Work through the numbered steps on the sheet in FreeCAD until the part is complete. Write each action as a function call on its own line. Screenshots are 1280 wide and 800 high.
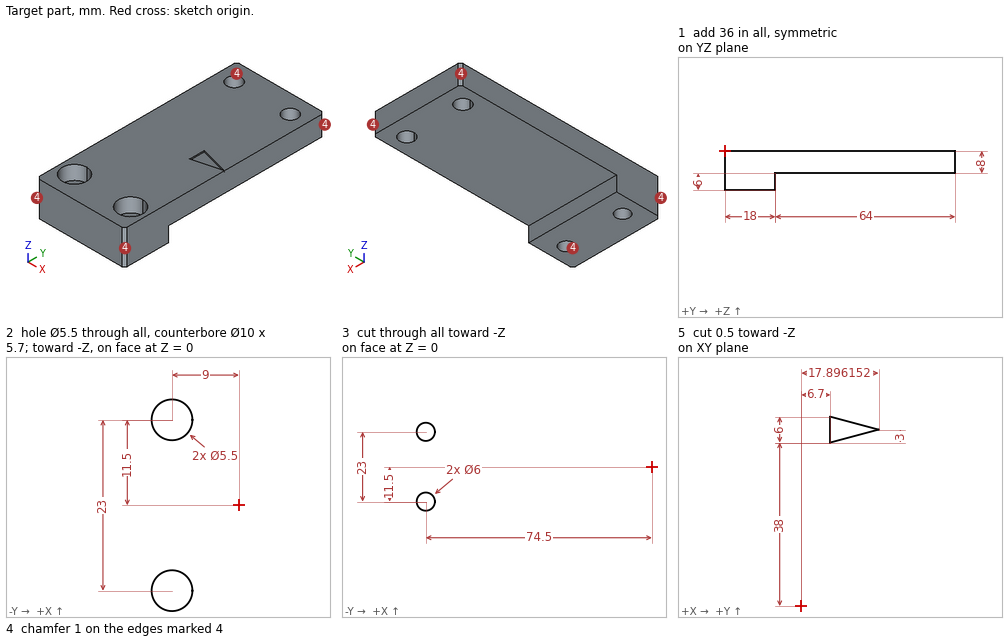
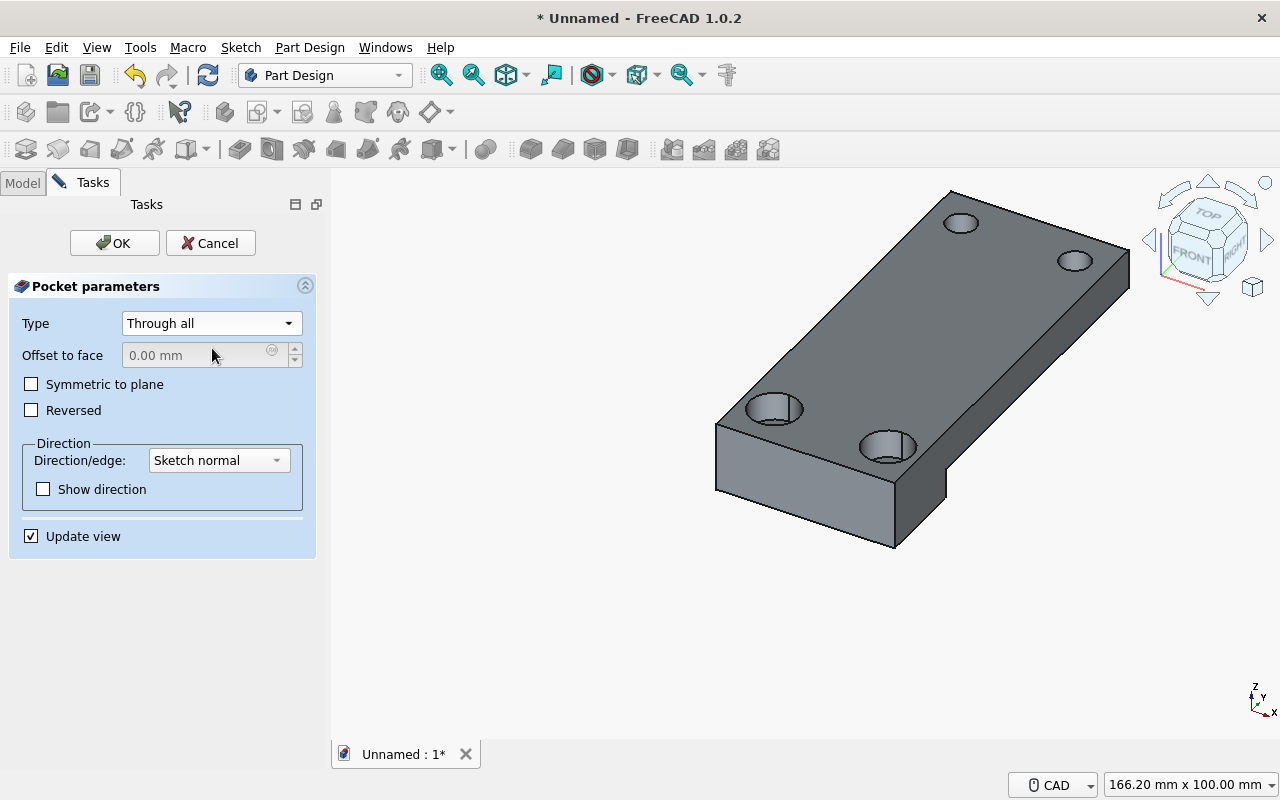
click(115, 243)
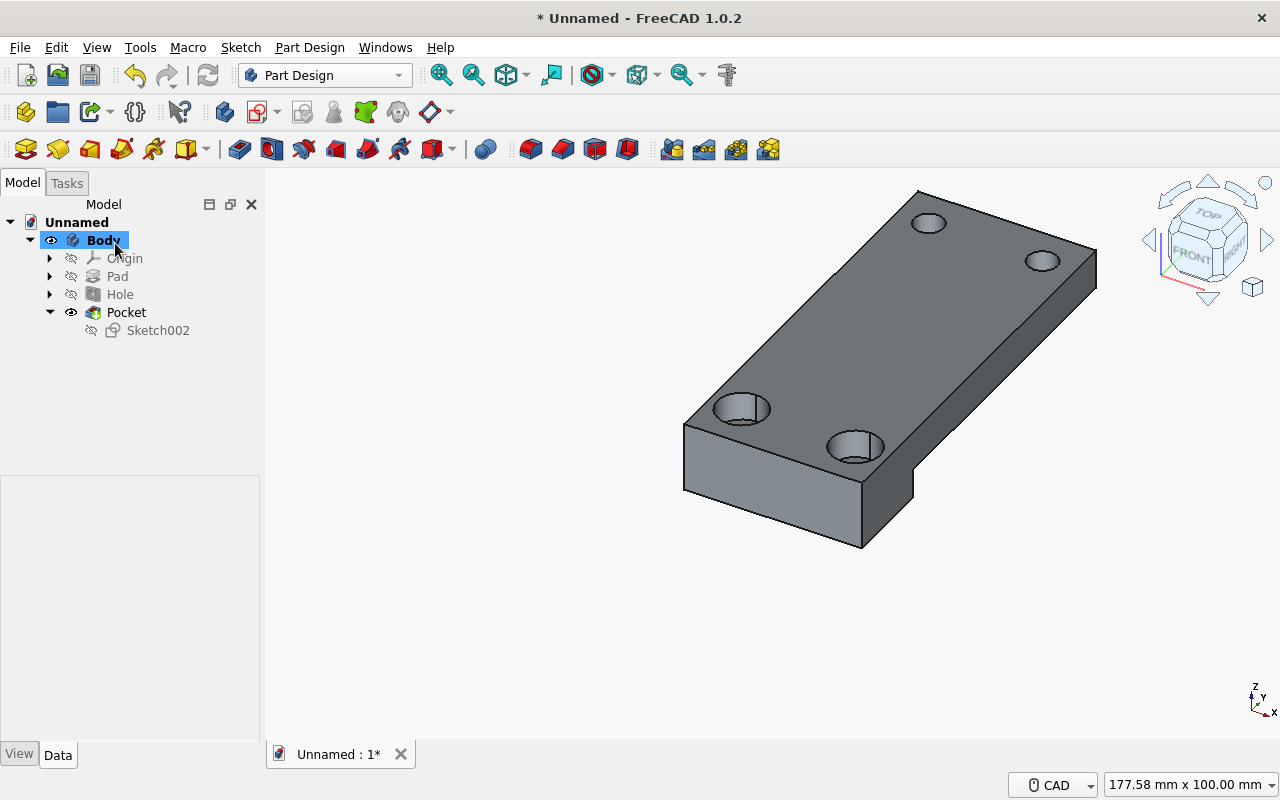
click(862, 515)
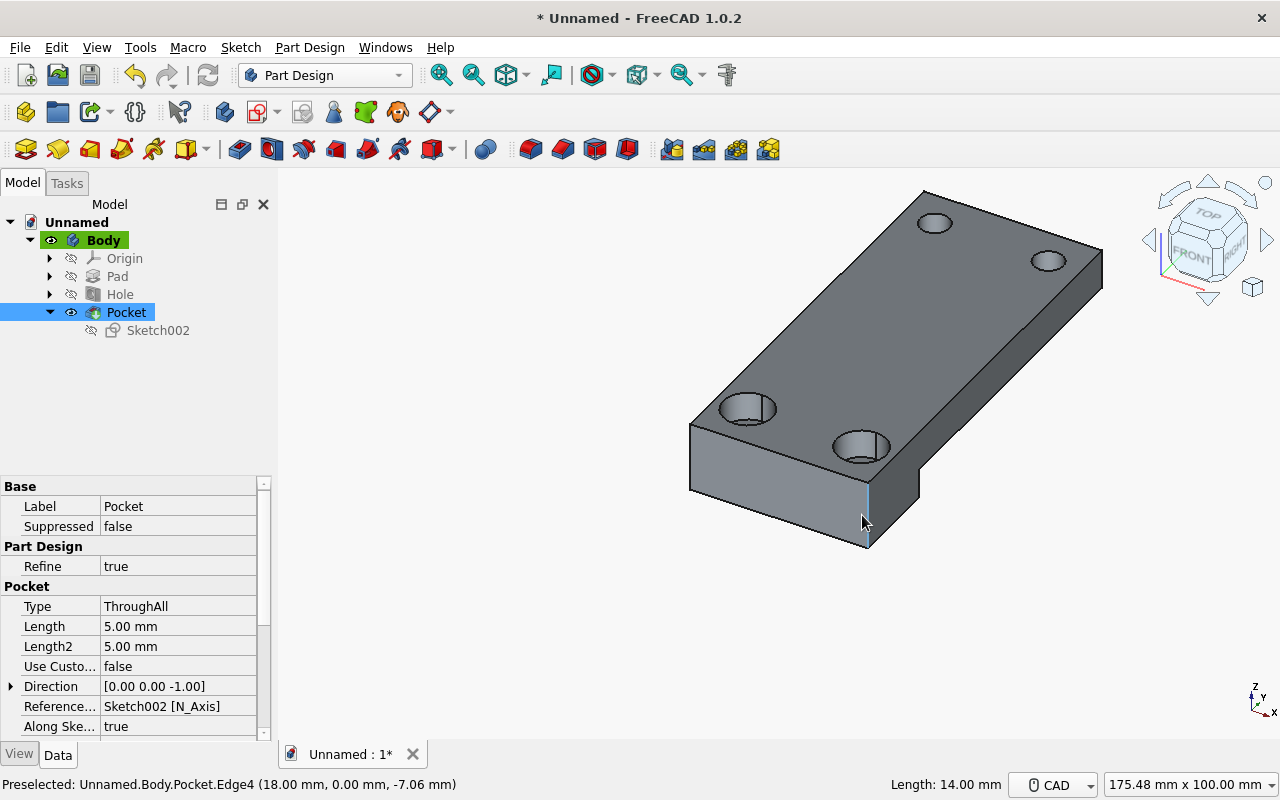
key(0)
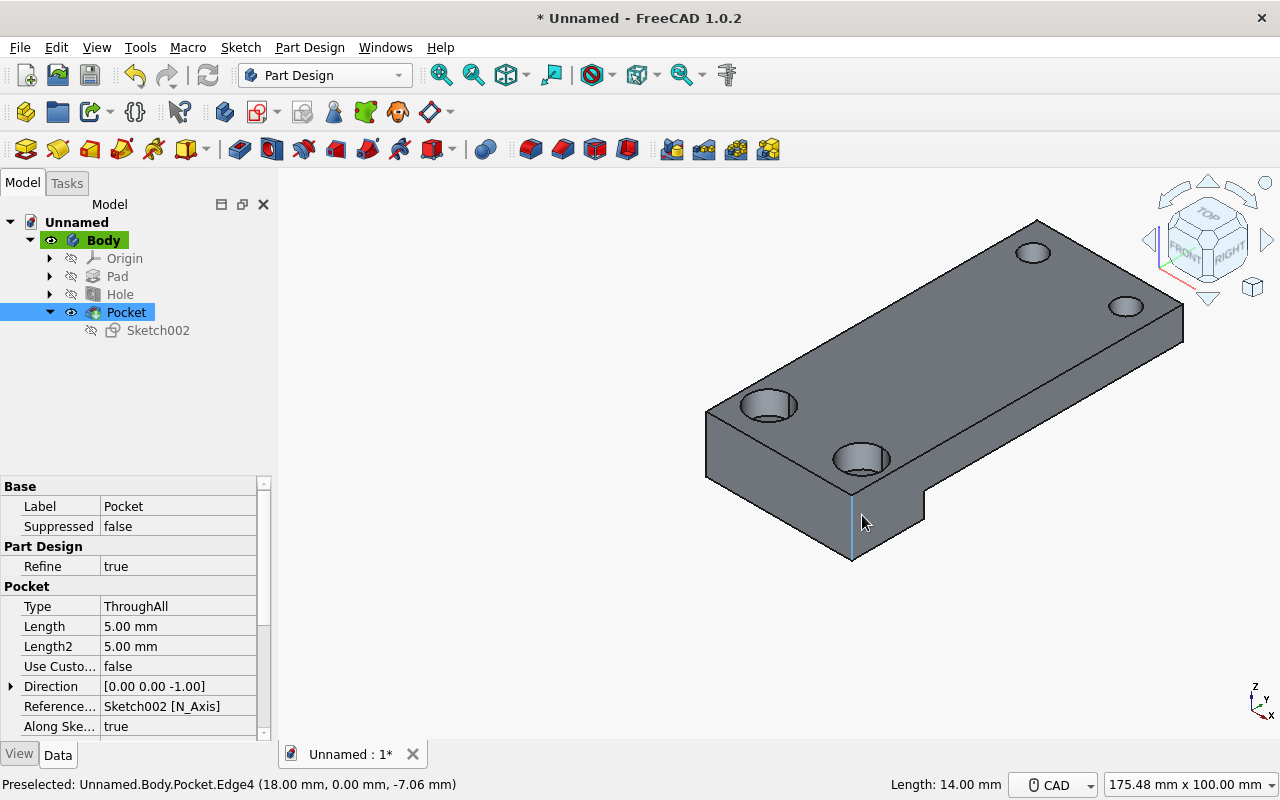
key(2)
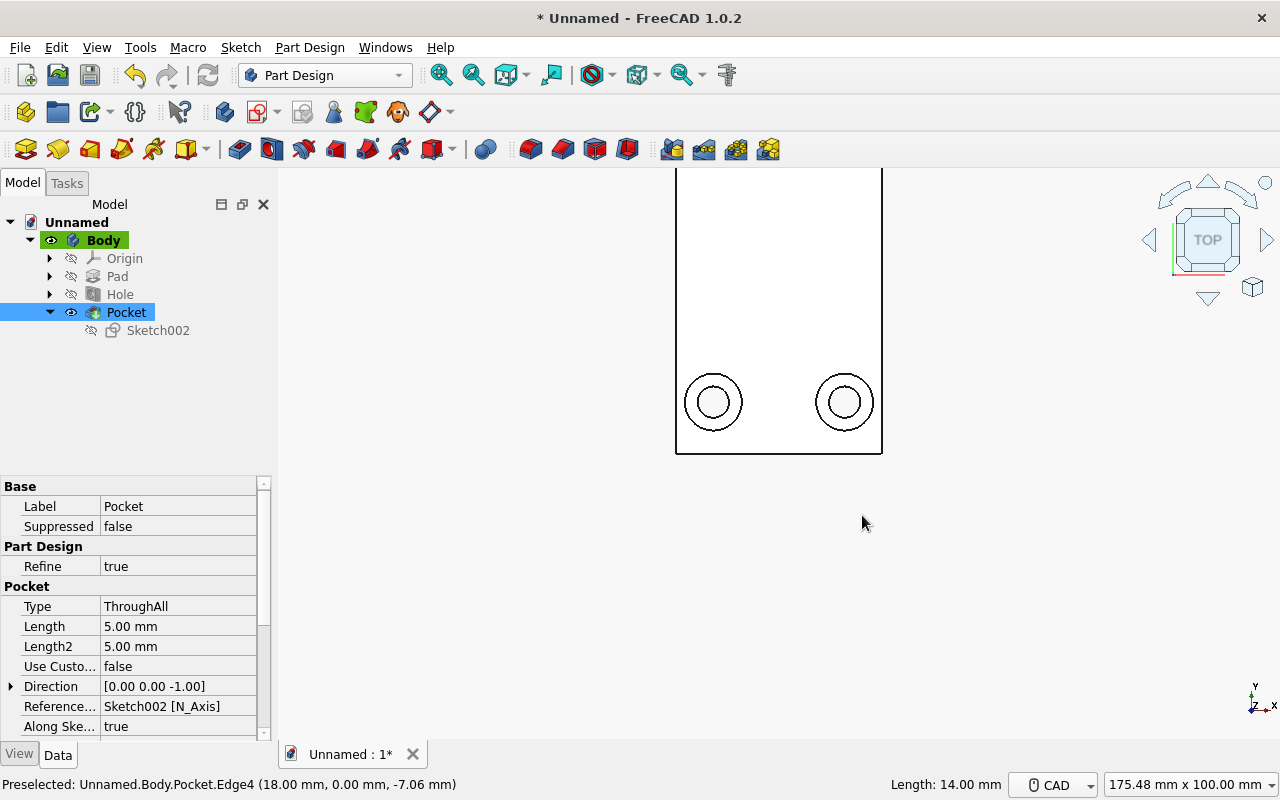
click(442, 76)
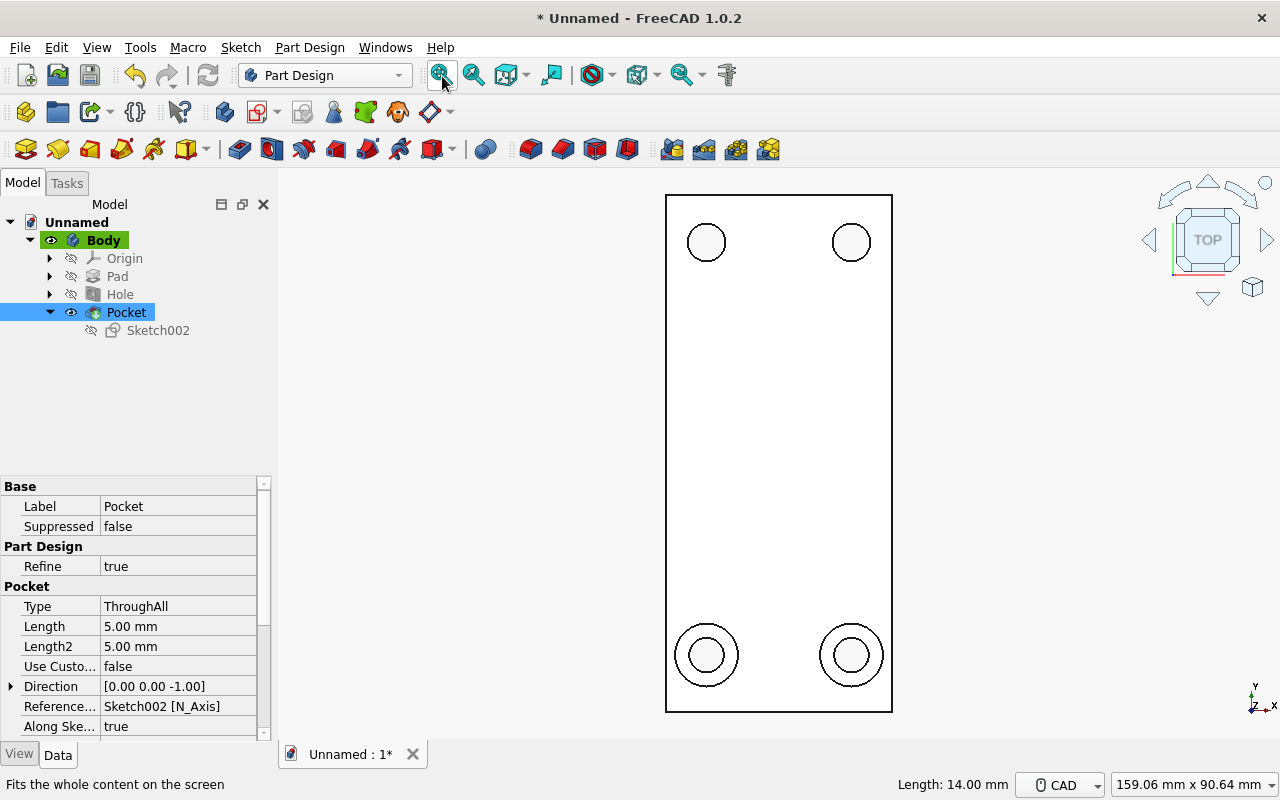
key(1)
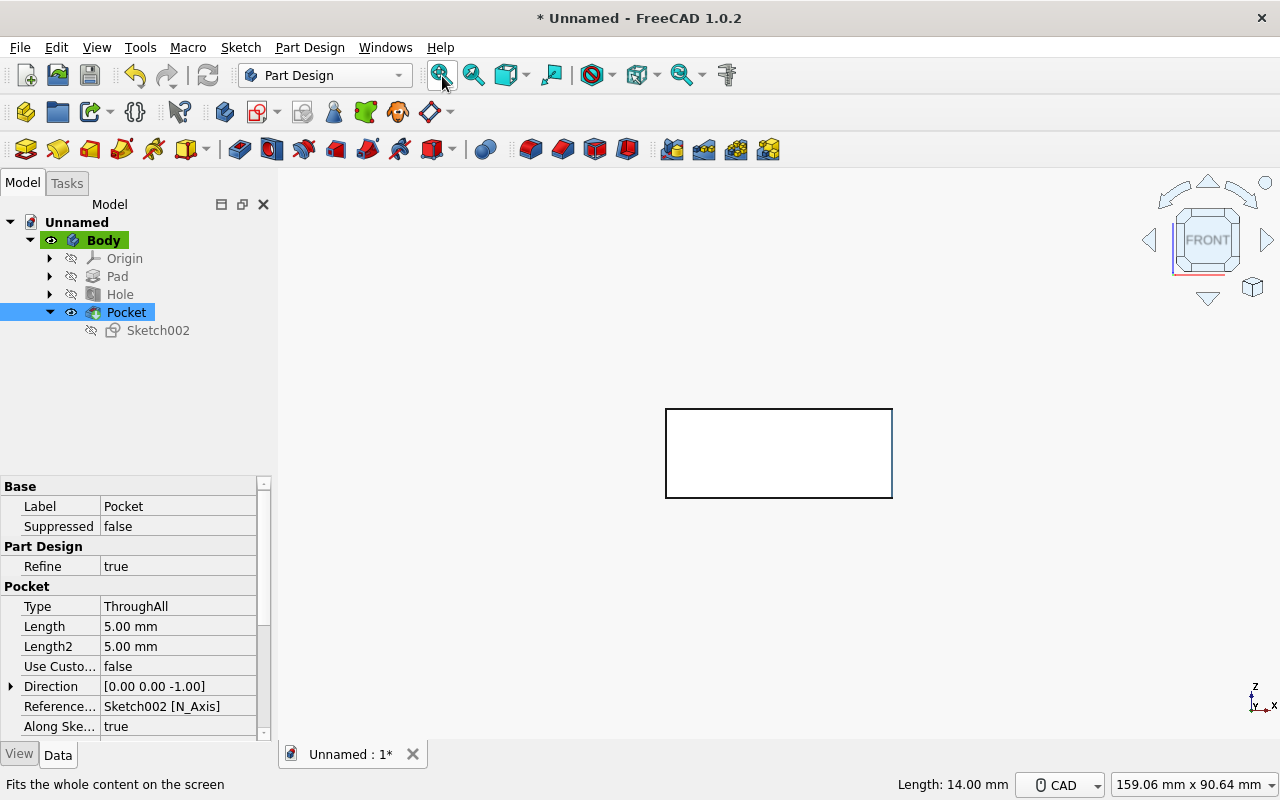
click(442, 76)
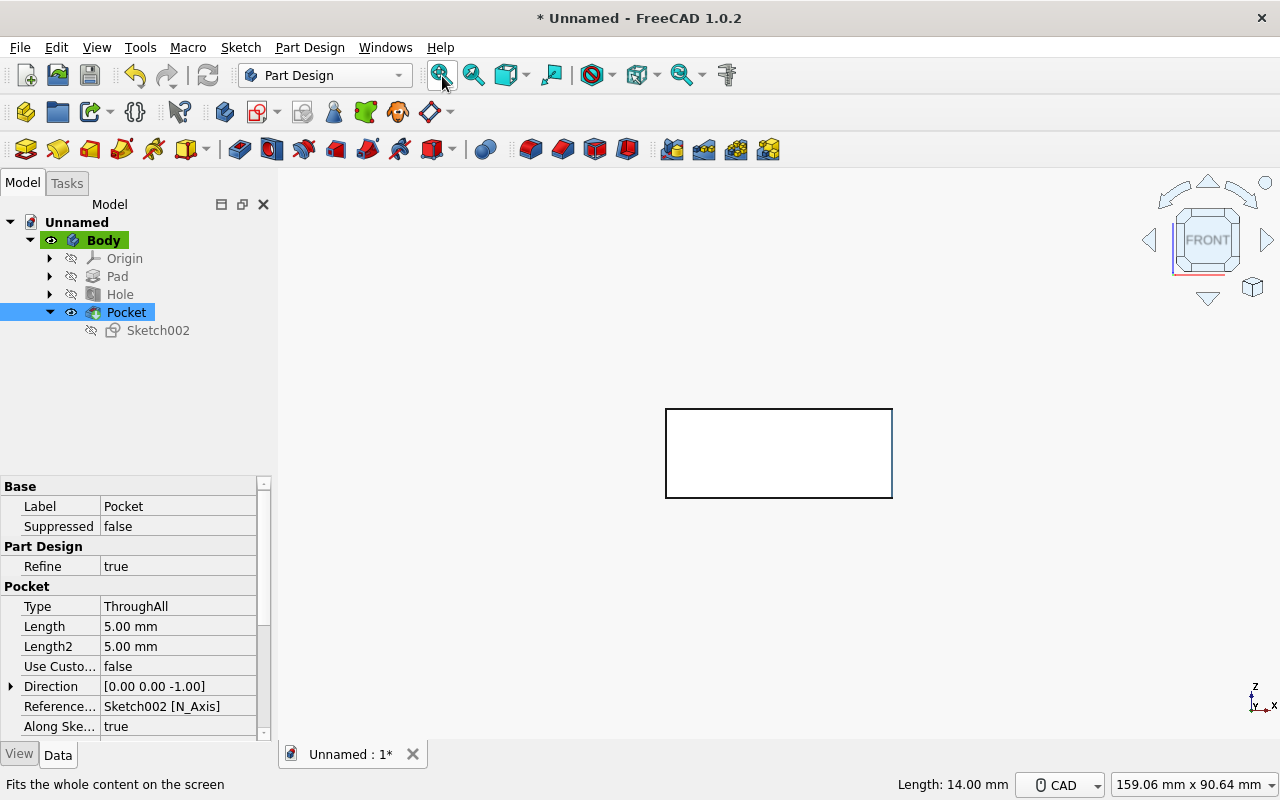
key(3)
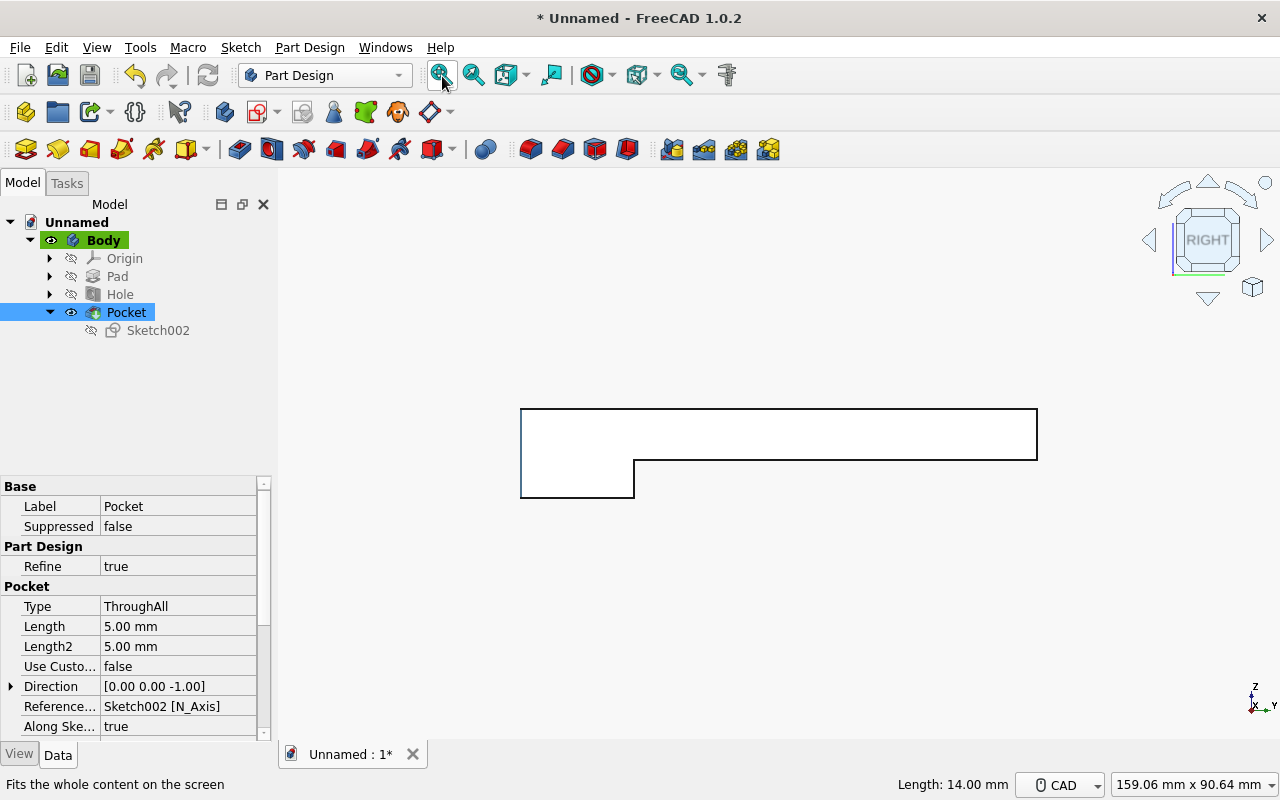
click(1037, 434, ctrl)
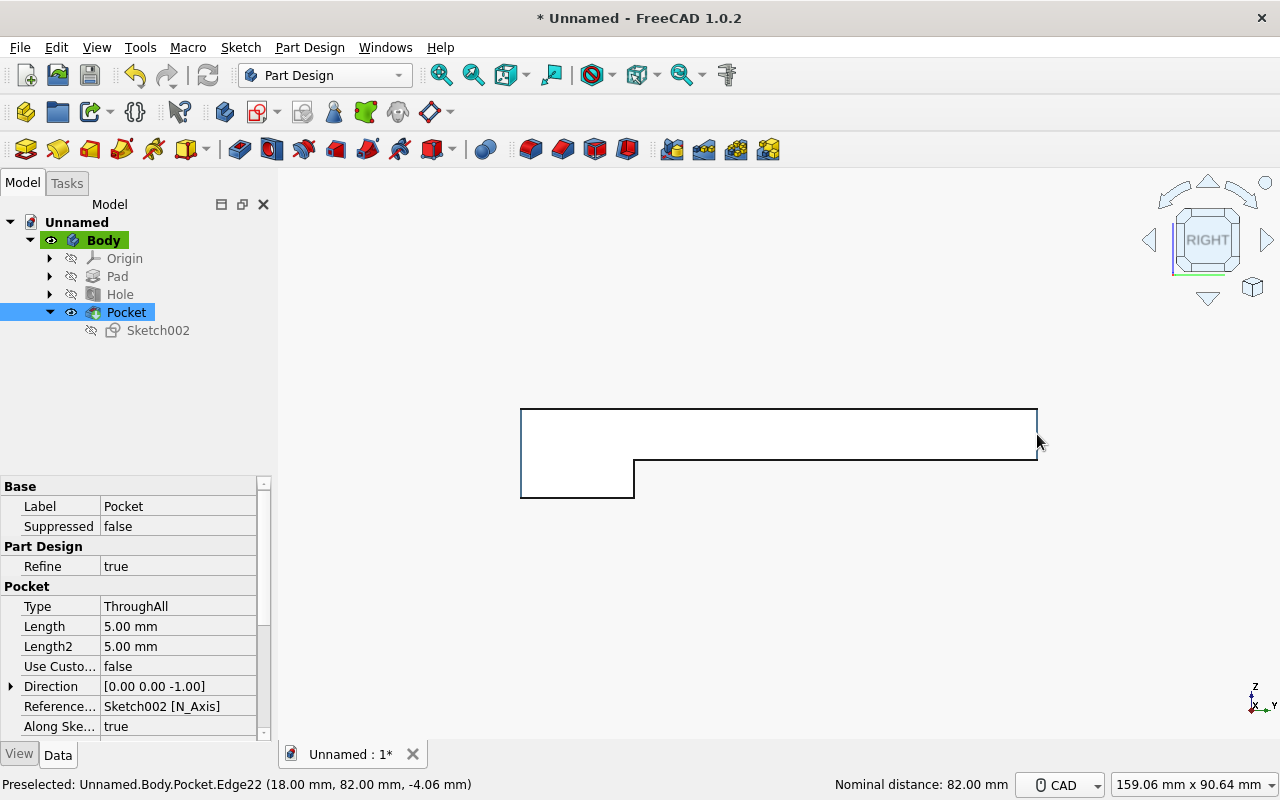
key(5)